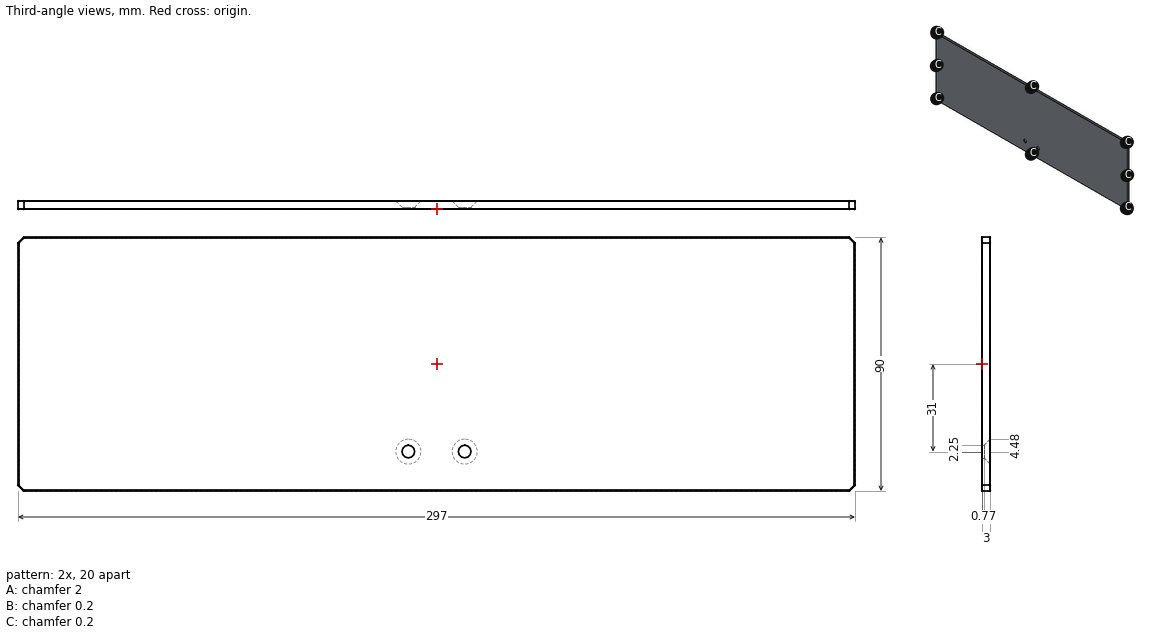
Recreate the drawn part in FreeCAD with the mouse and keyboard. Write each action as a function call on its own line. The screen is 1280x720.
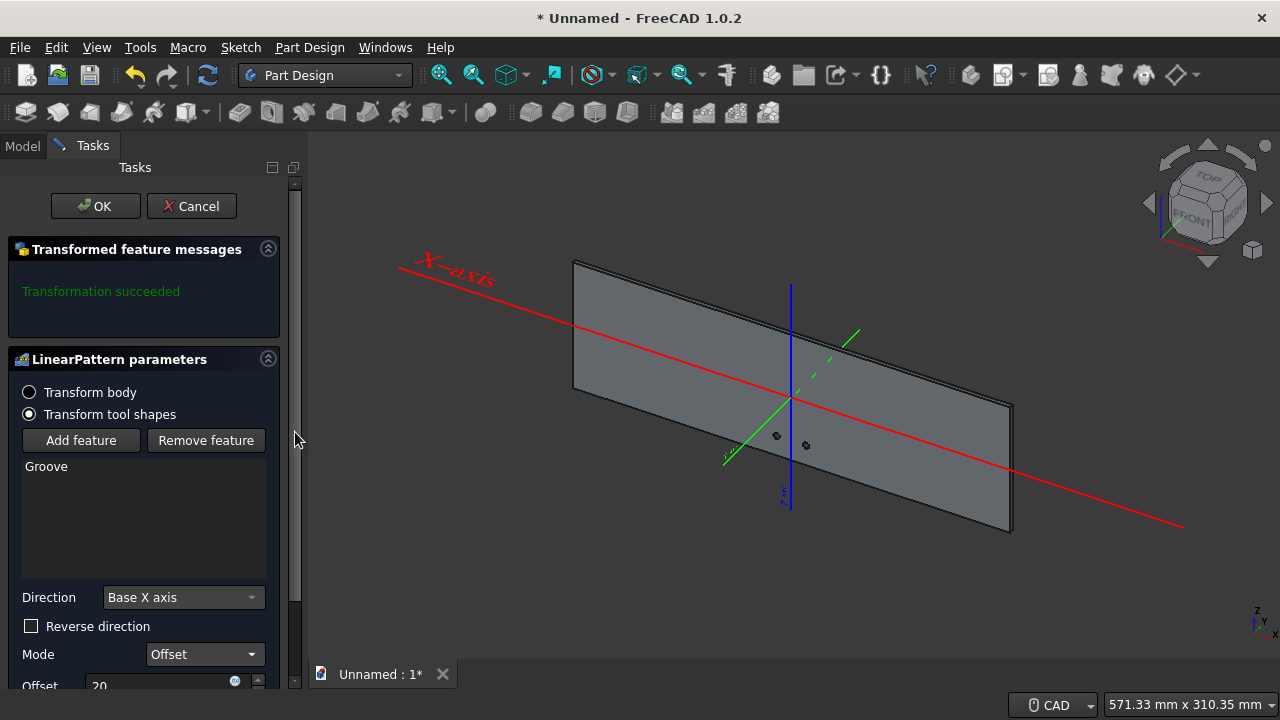
click(96, 206)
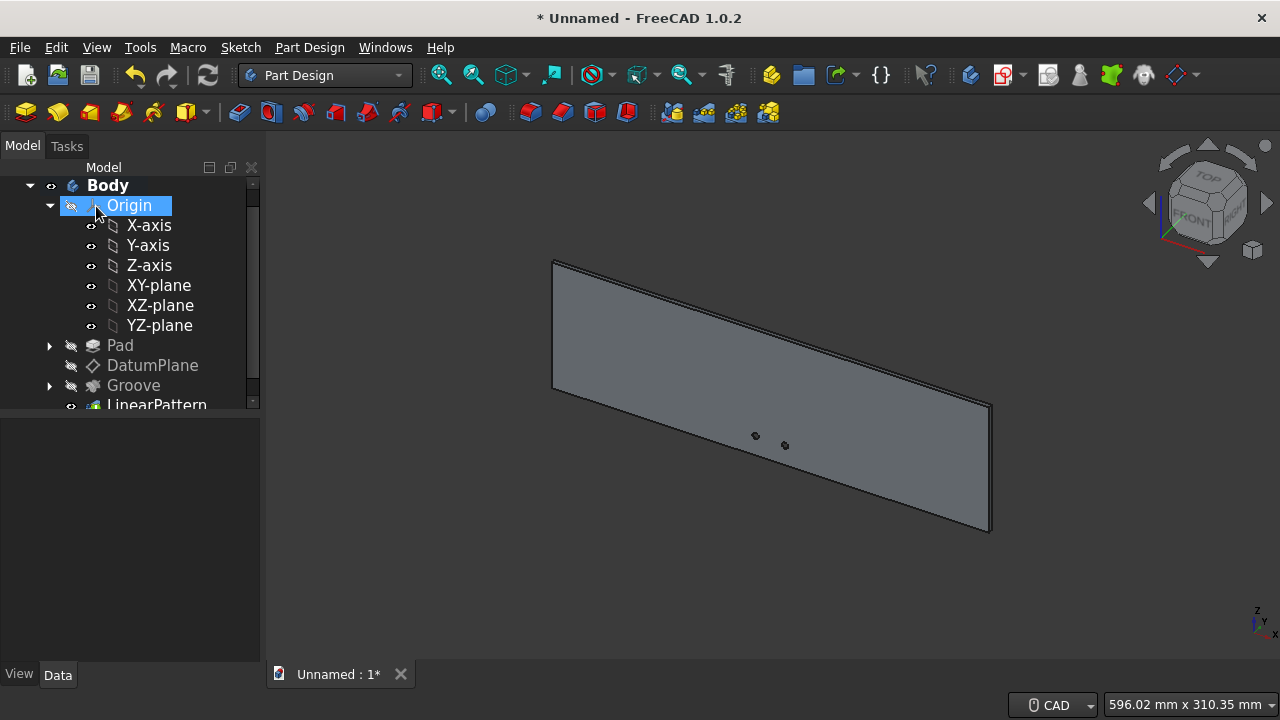
scroll(990, 405, up, 11)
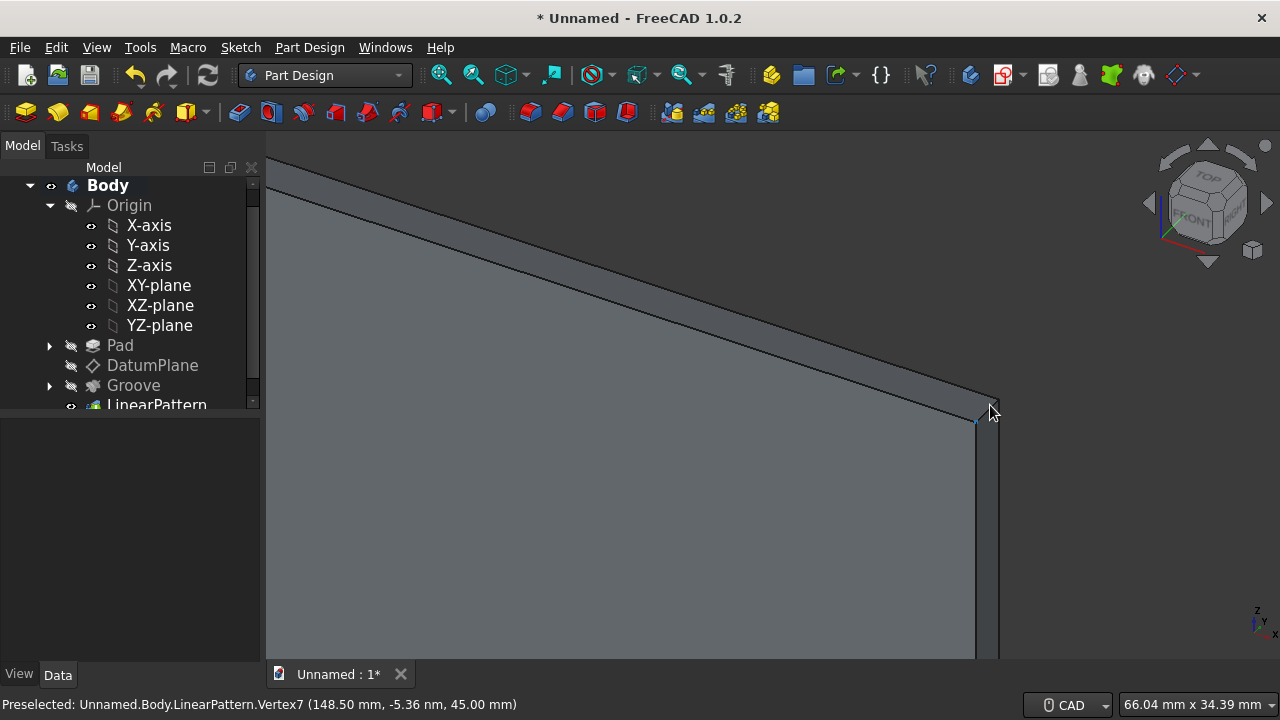
click(988, 410)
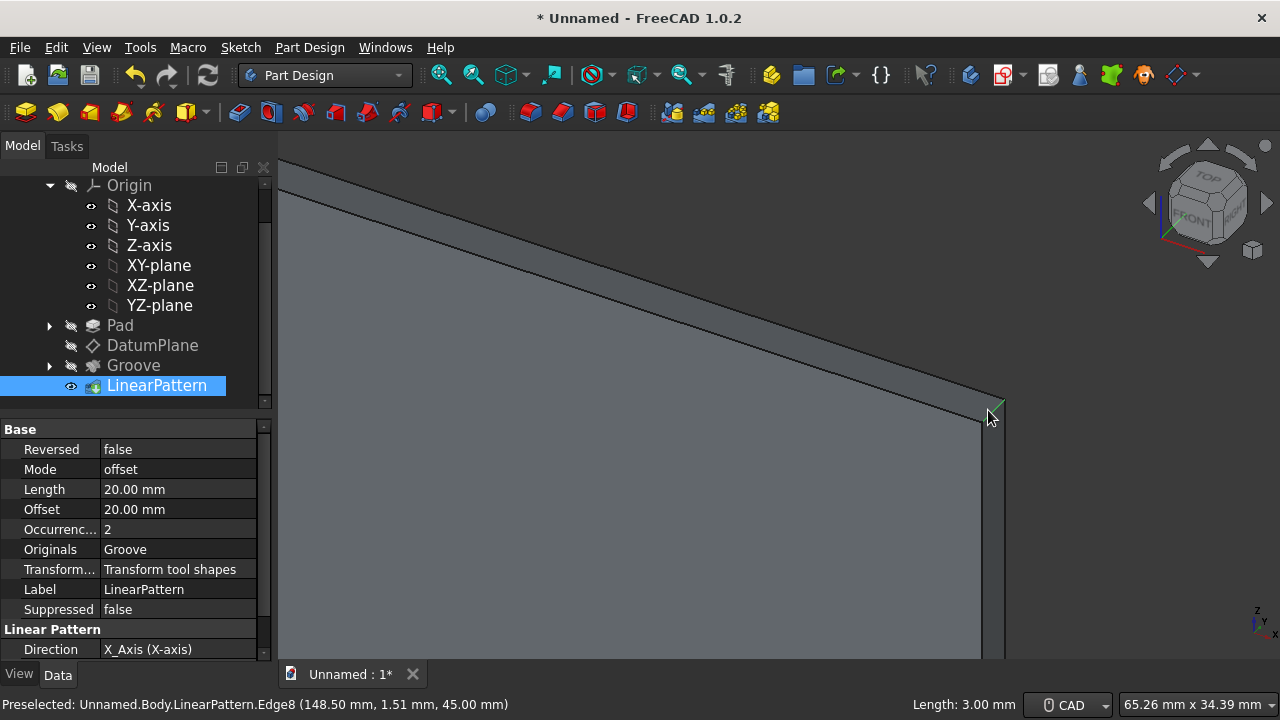
key(v)
key(f)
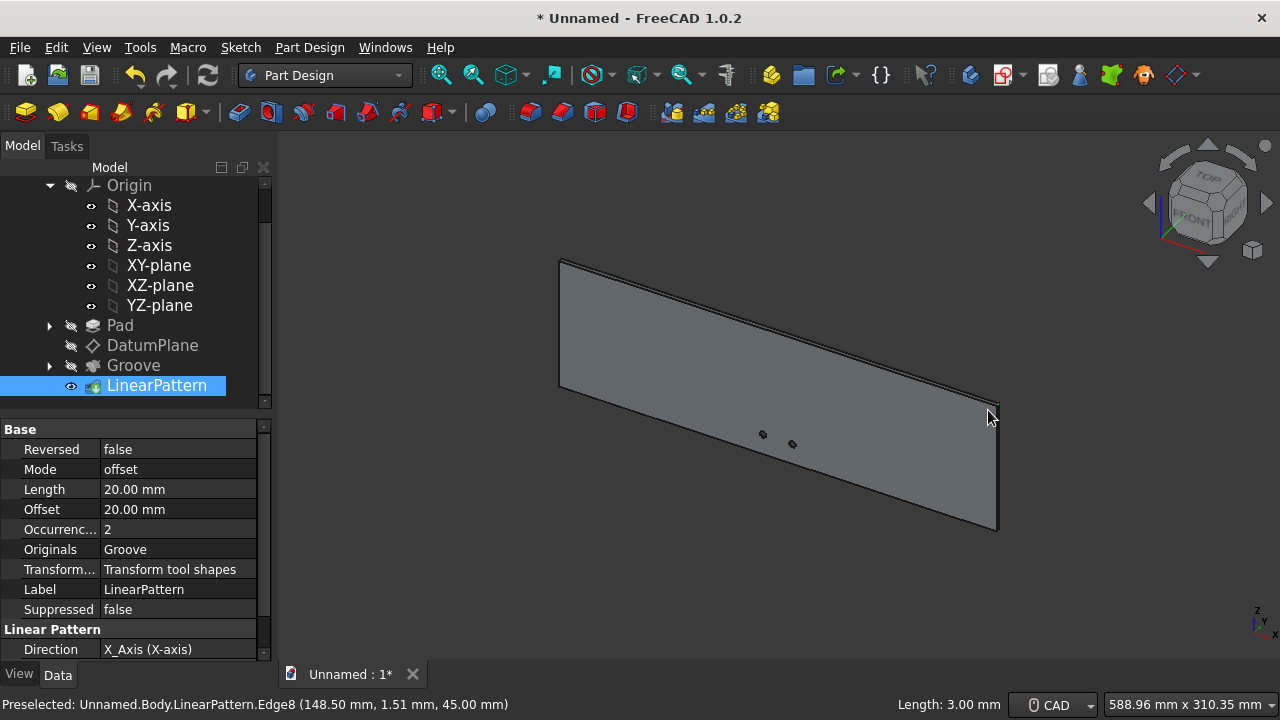
key(0)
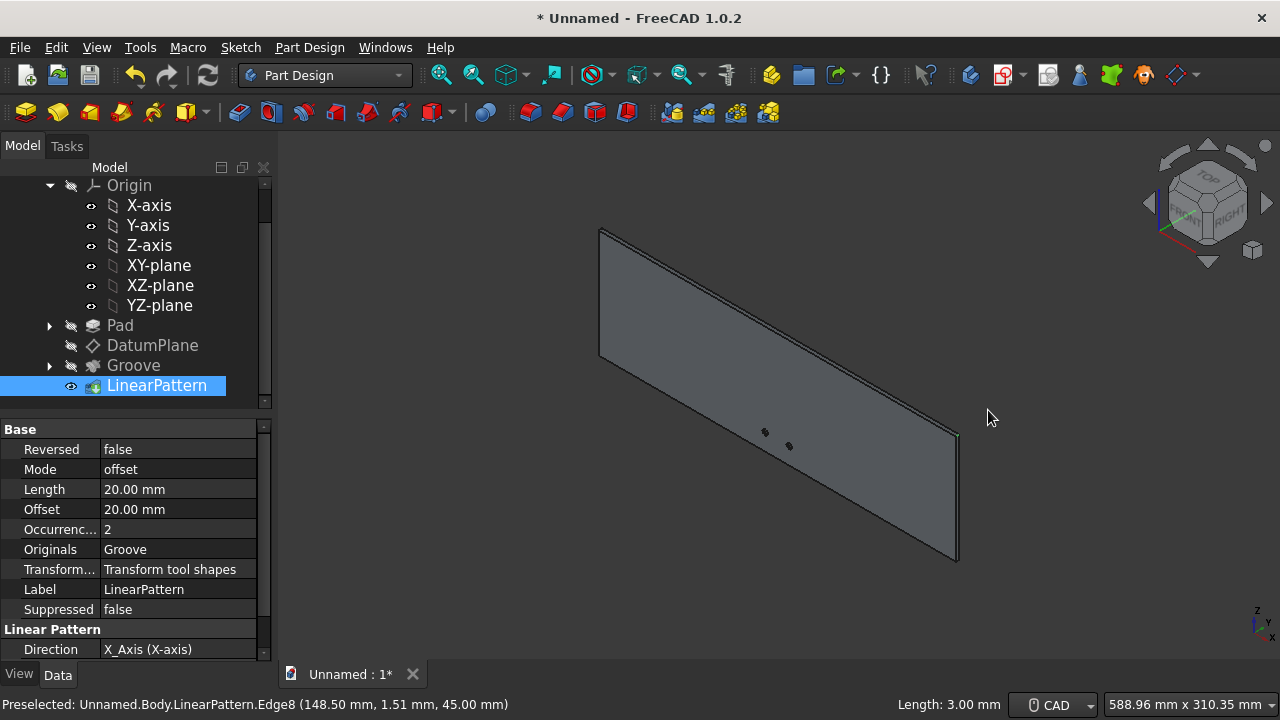
scroll(600, 228, up, 11)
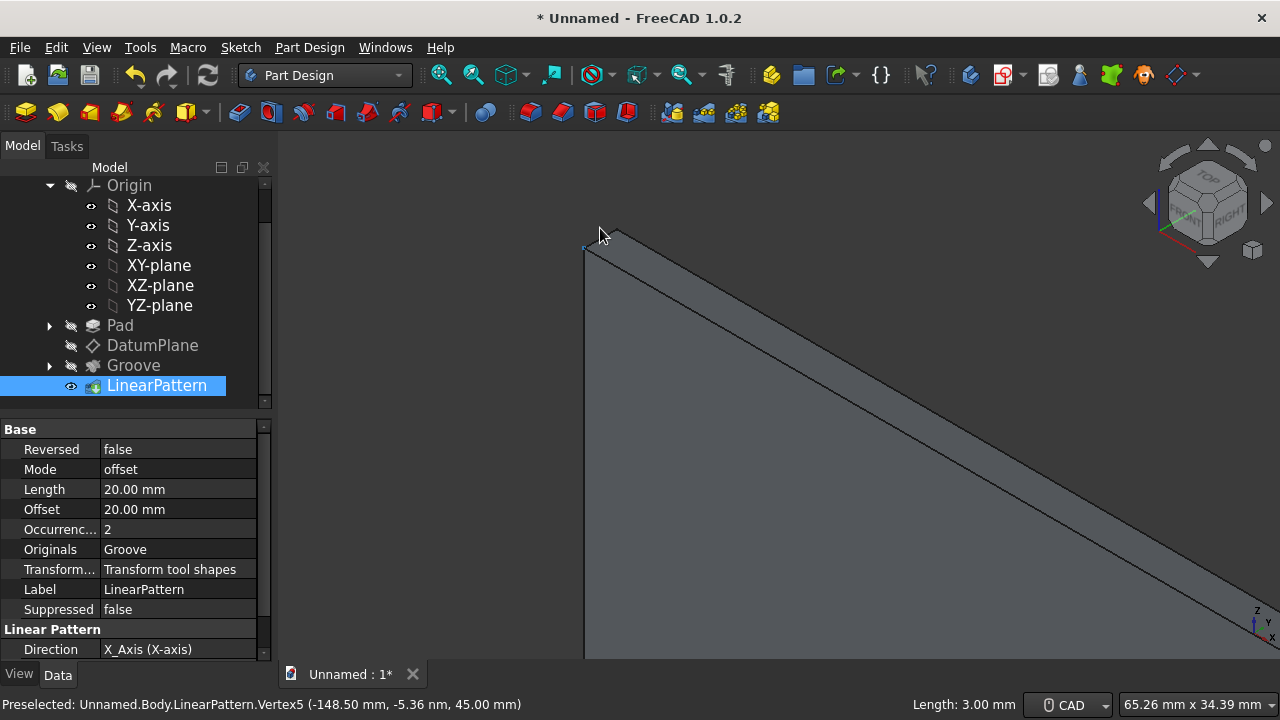
click(442, 76)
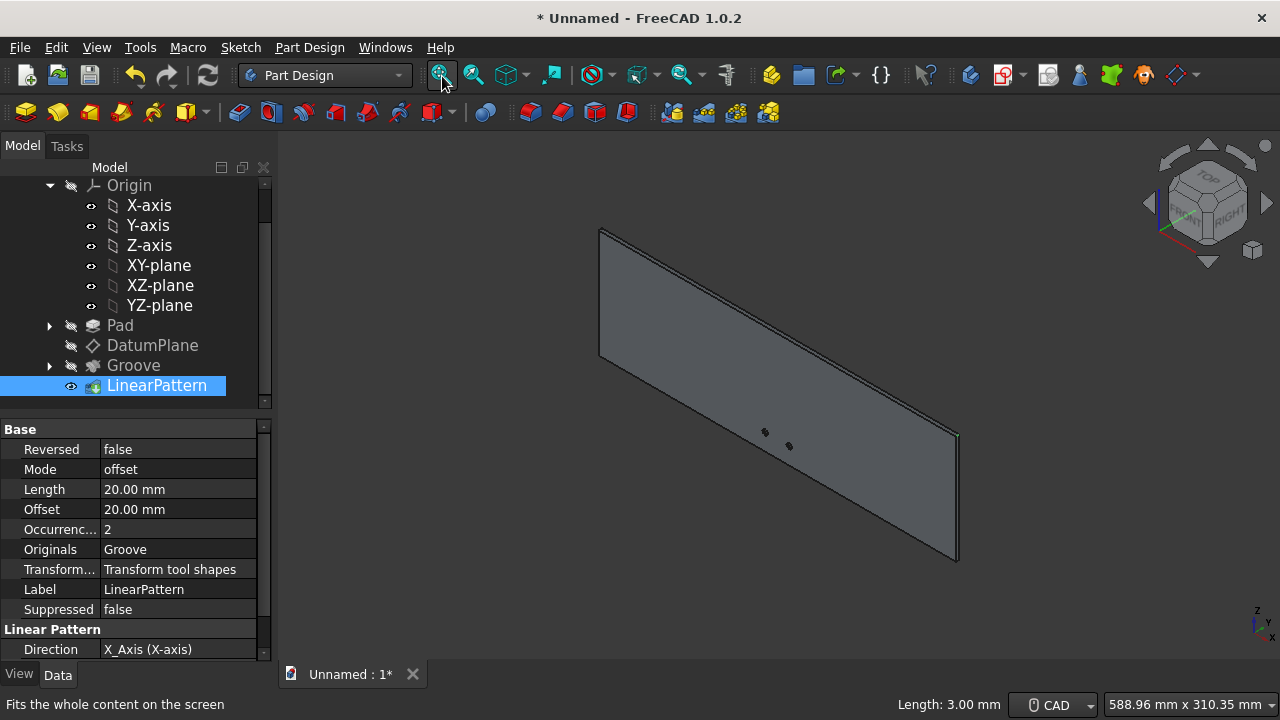
key(2)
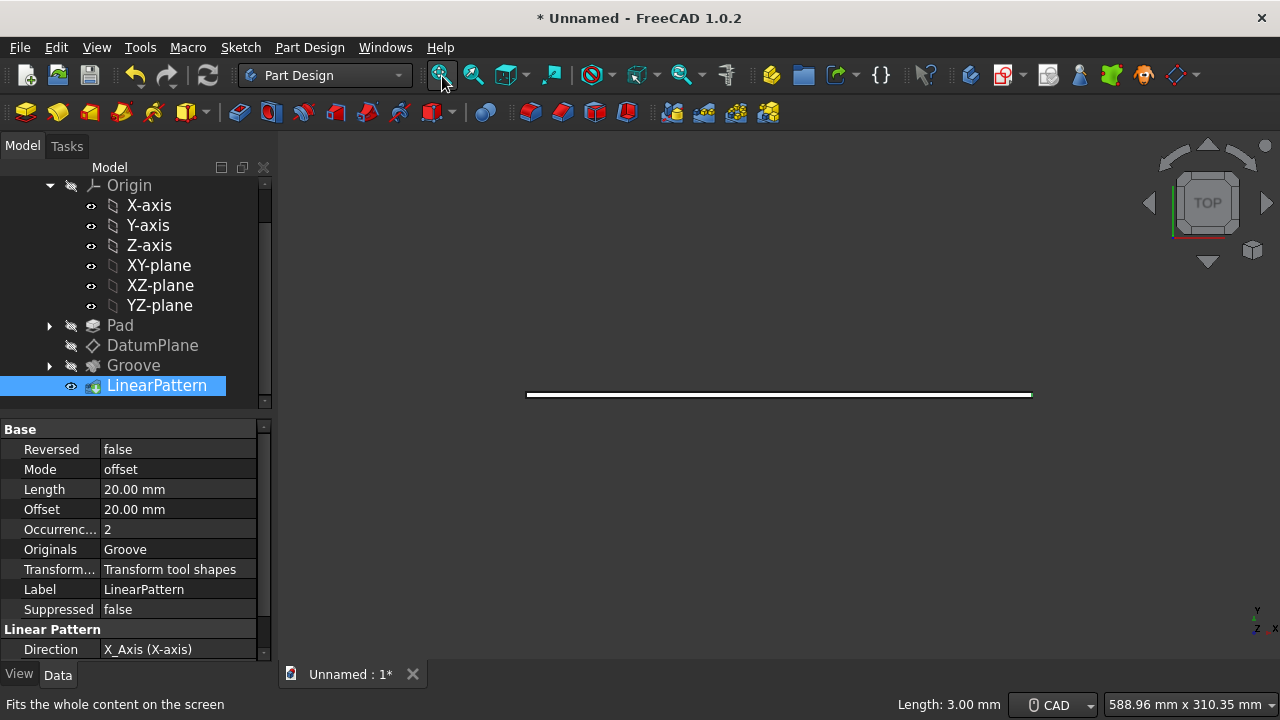
scroll(526, 394, up, 11)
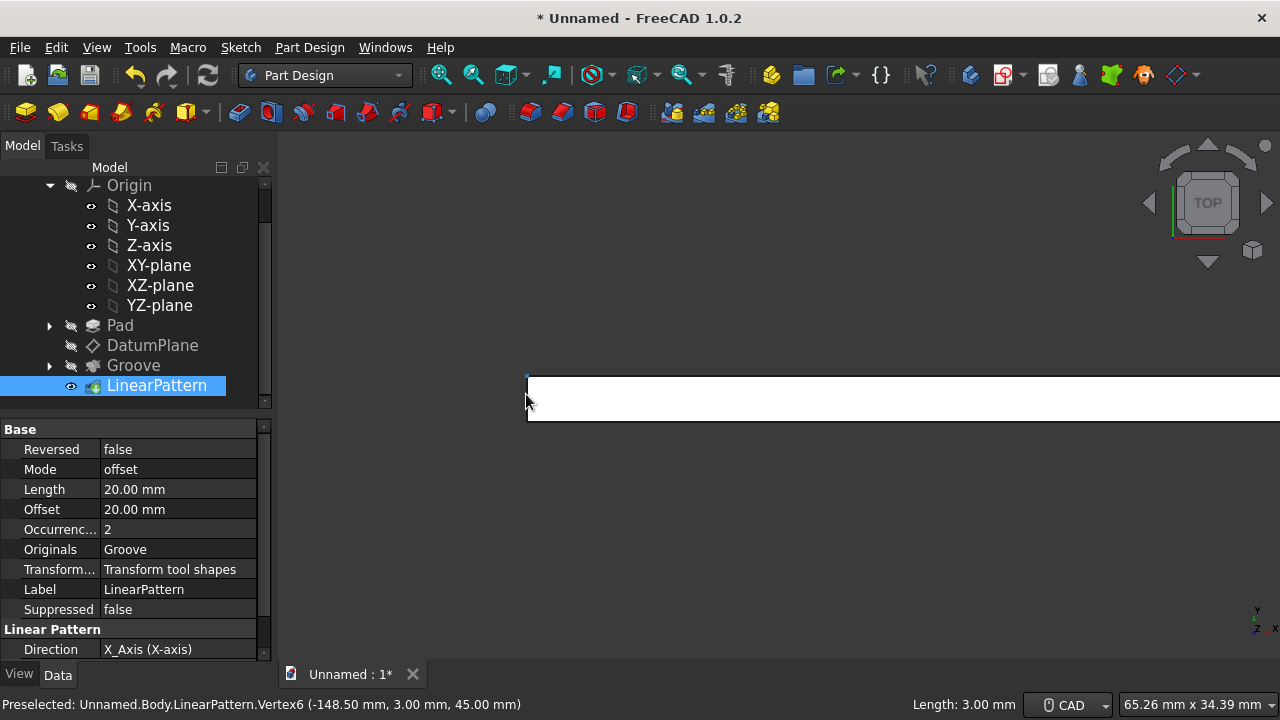
click(527, 398, ctrl)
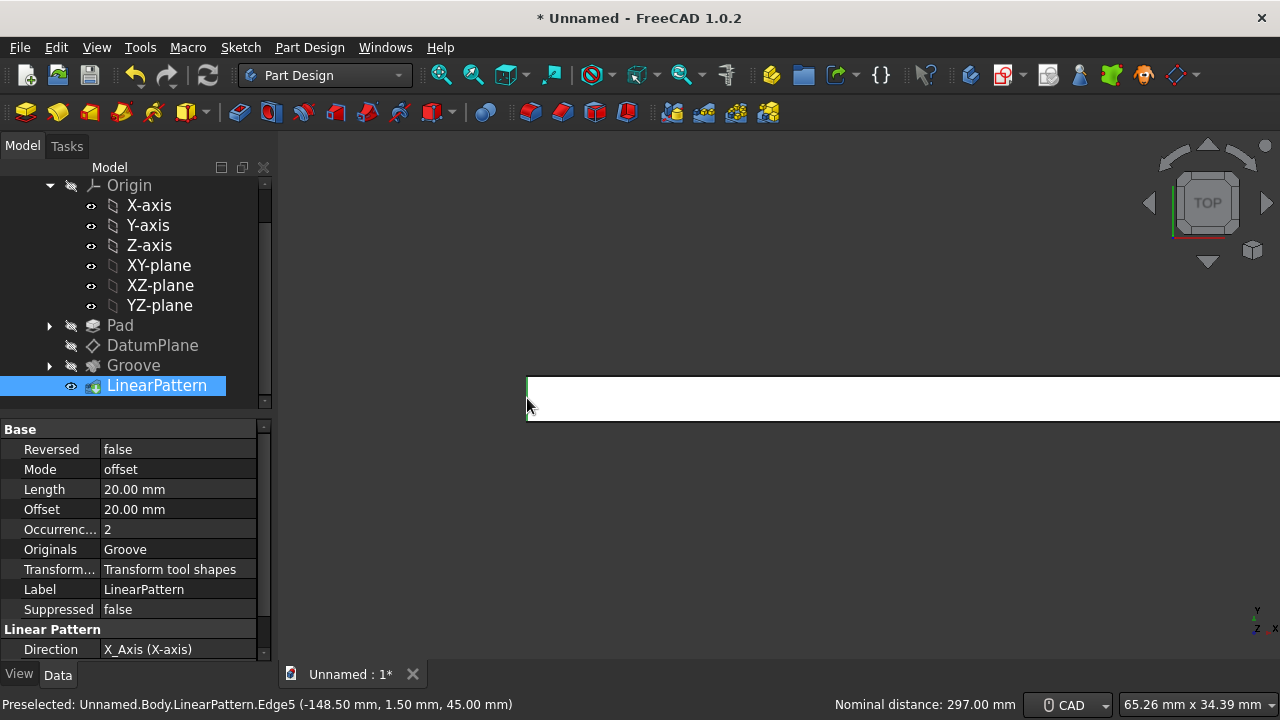
key(v)
key(f)